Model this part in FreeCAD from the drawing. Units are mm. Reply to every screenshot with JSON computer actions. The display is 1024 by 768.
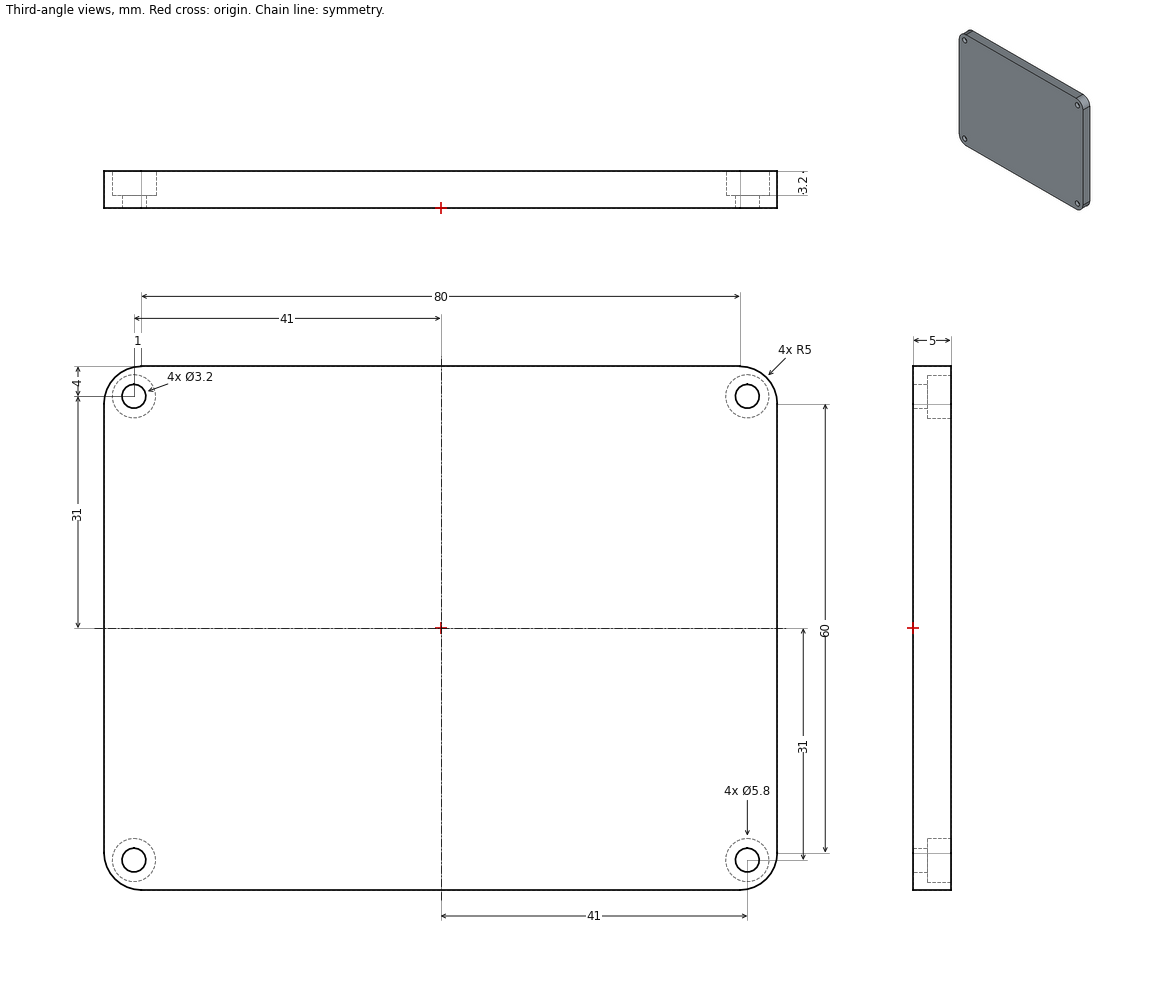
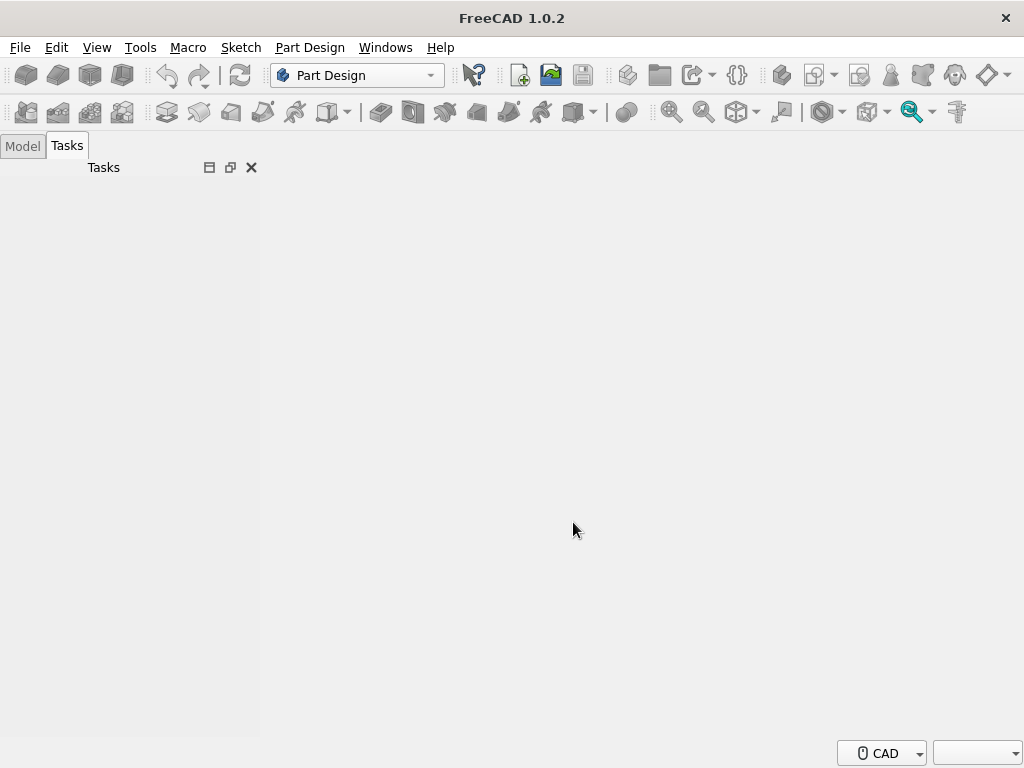
{"action": "key", "text": "ctrl+n"}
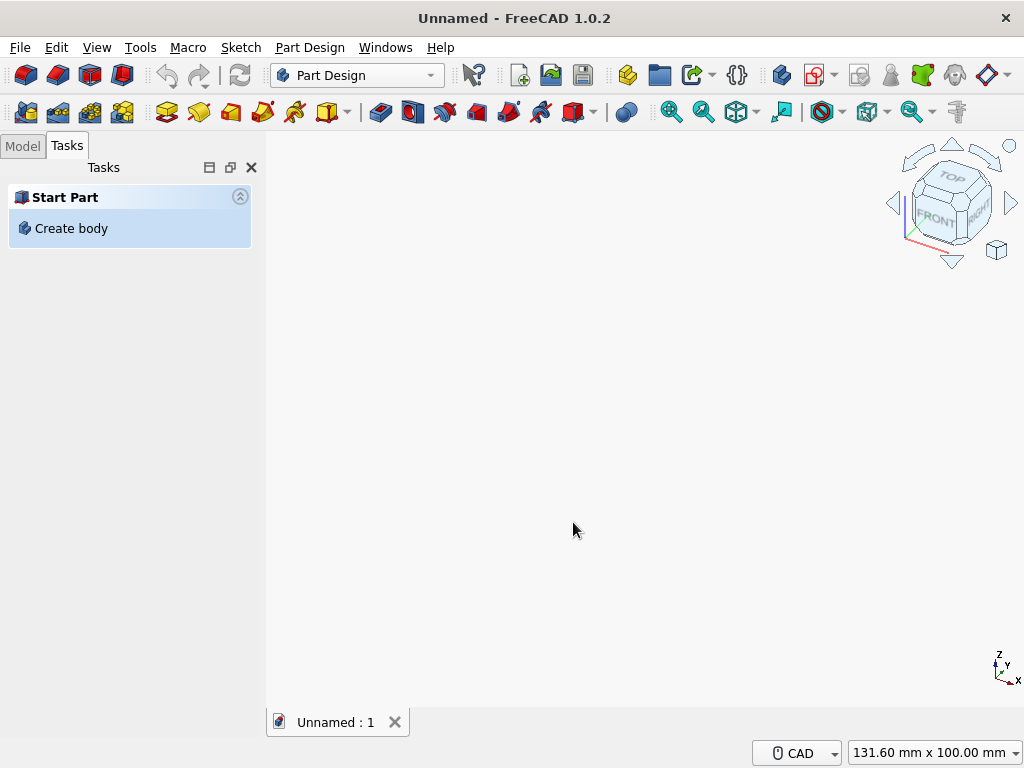
{"action": "left_click", "coordinate": [814, 76]}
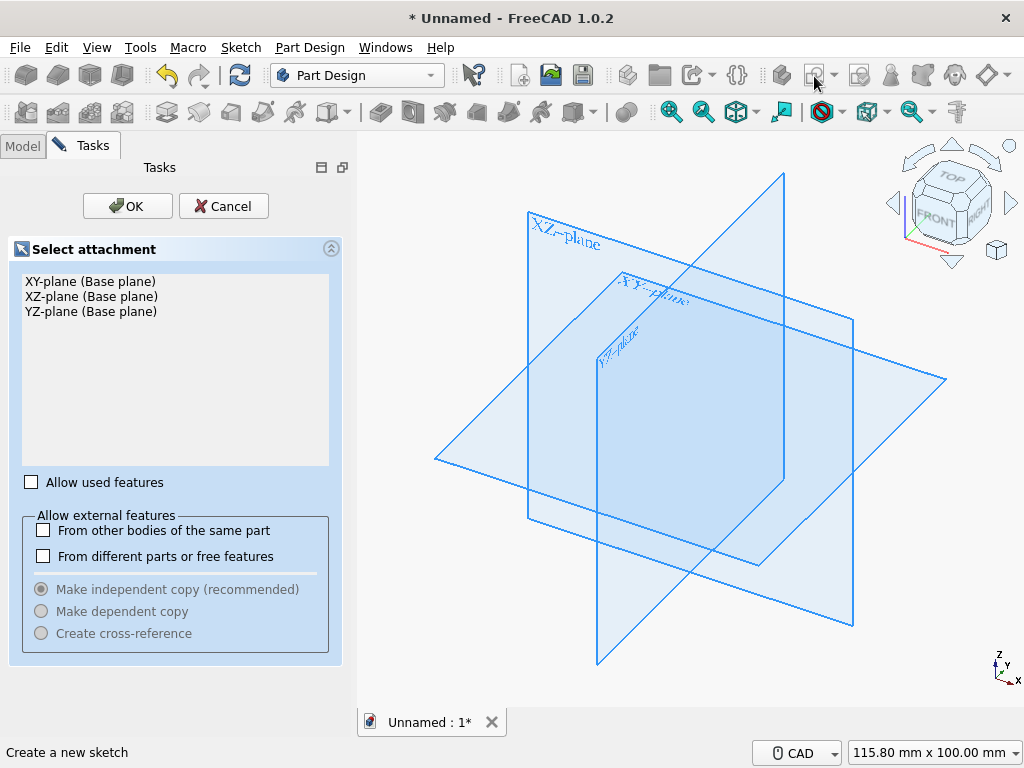
{"action": "left_click", "coordinate": [82, 296]}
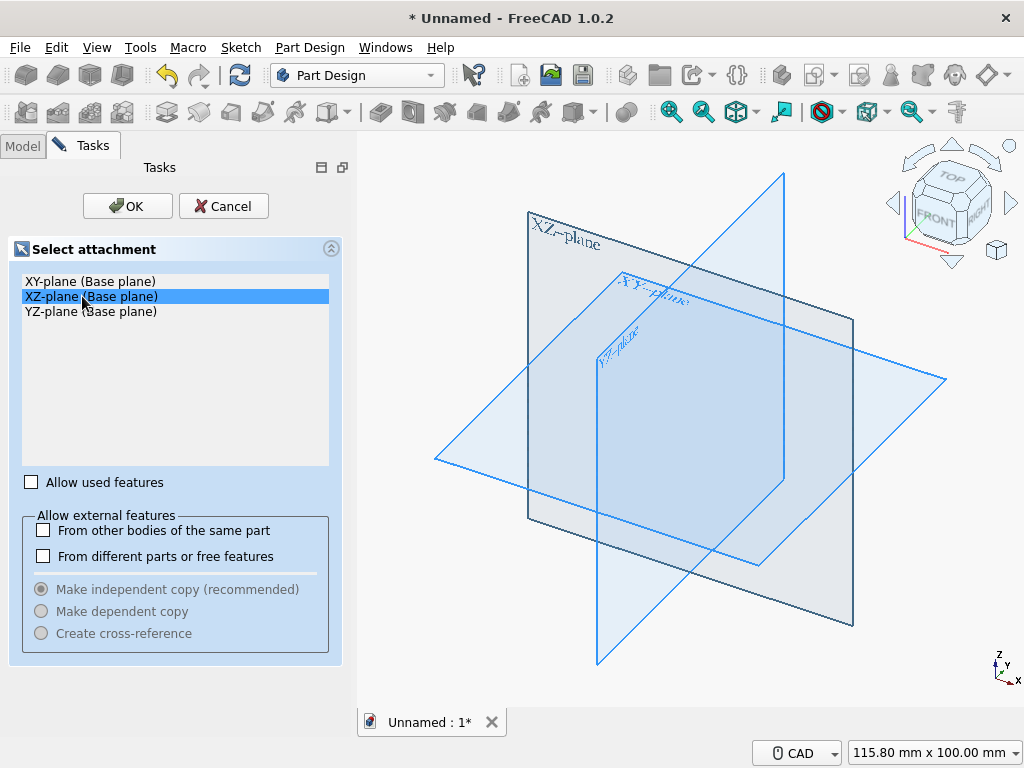
{"action": "left_click", "coordinate": [128, 206]}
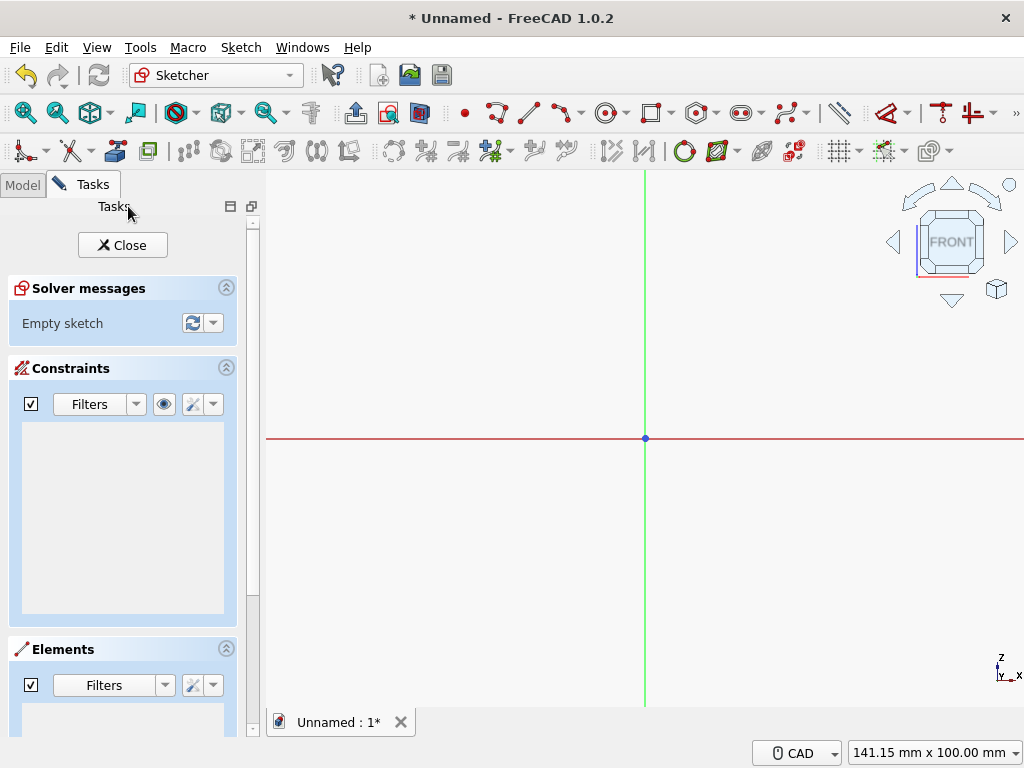
{"action": "scroll", "coordinate": [294, 439], "scroll_direction": "down", "scroll_amount": 1}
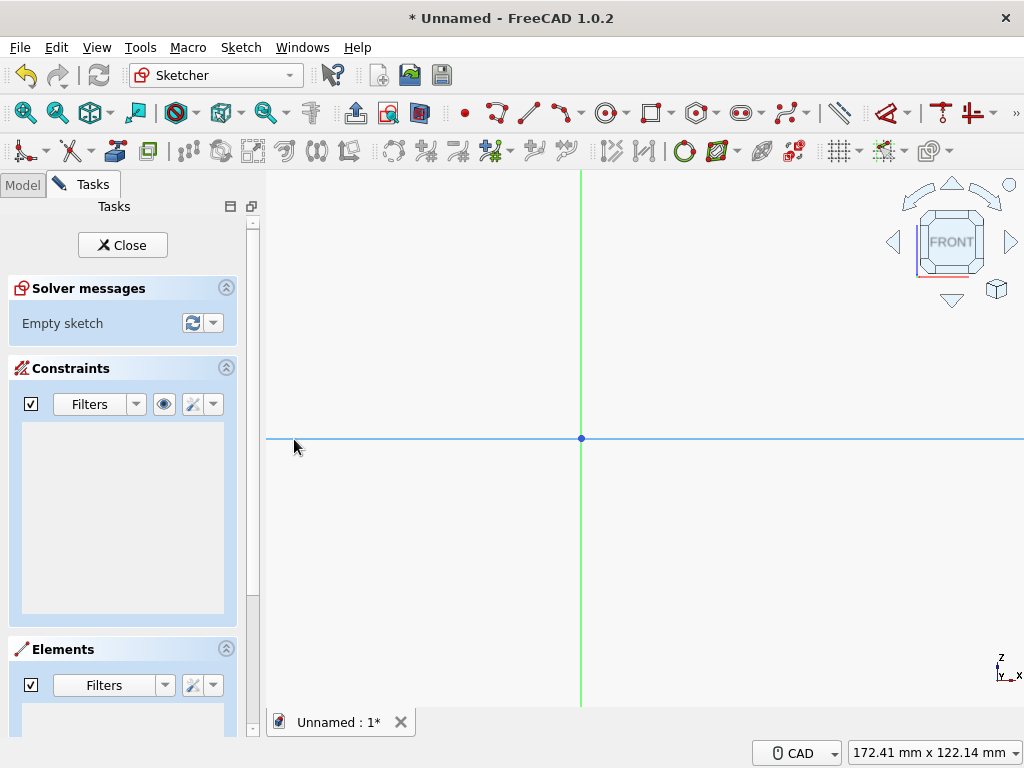
{"action": "key", "text": "g l"}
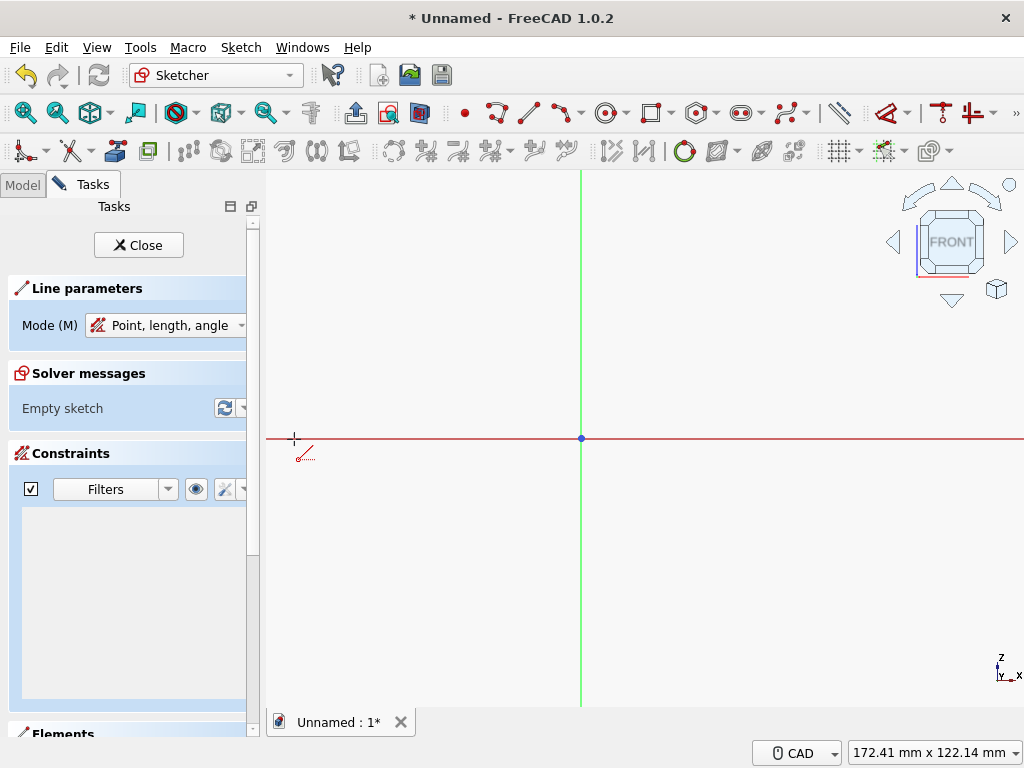
{"action": "left_click", "coordinate": [406, 285]}
{"action": "left_click", "coordinate": [757, 285]}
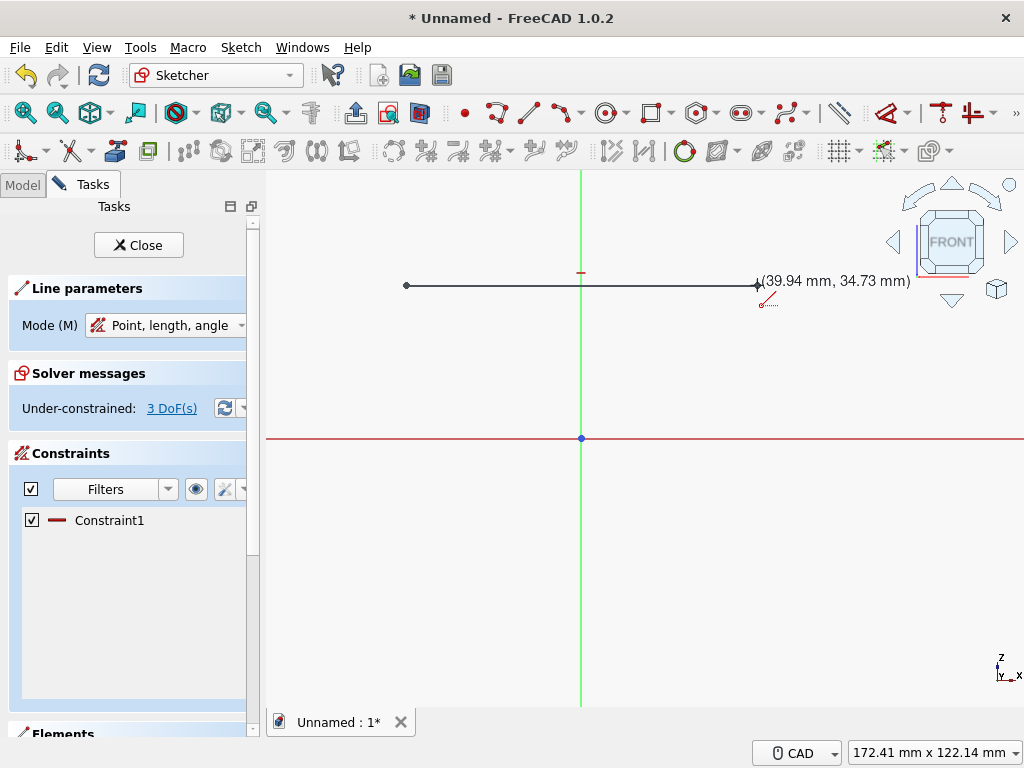
{"action": "left_click", "coordinate": [779, 307]}
{"action": "left_click", "coordinate": [779, 571]}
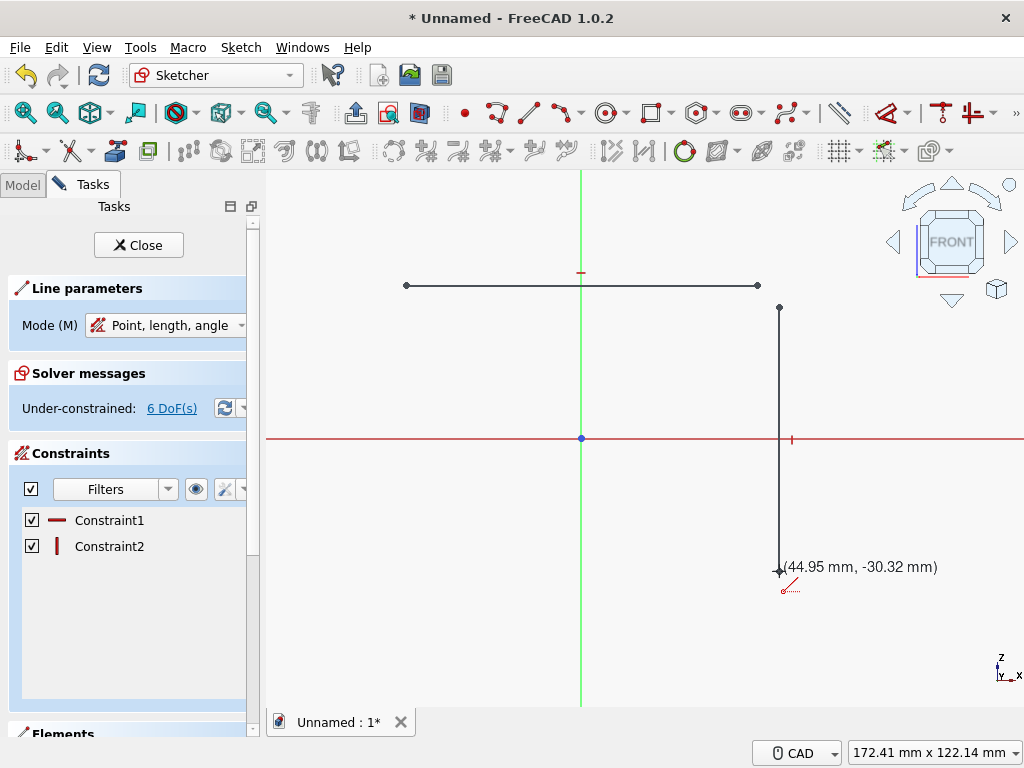
{"action": "left_click", "coordinate": [757, 593]}
{"action": "left_click", "coordinate": [406, 593]}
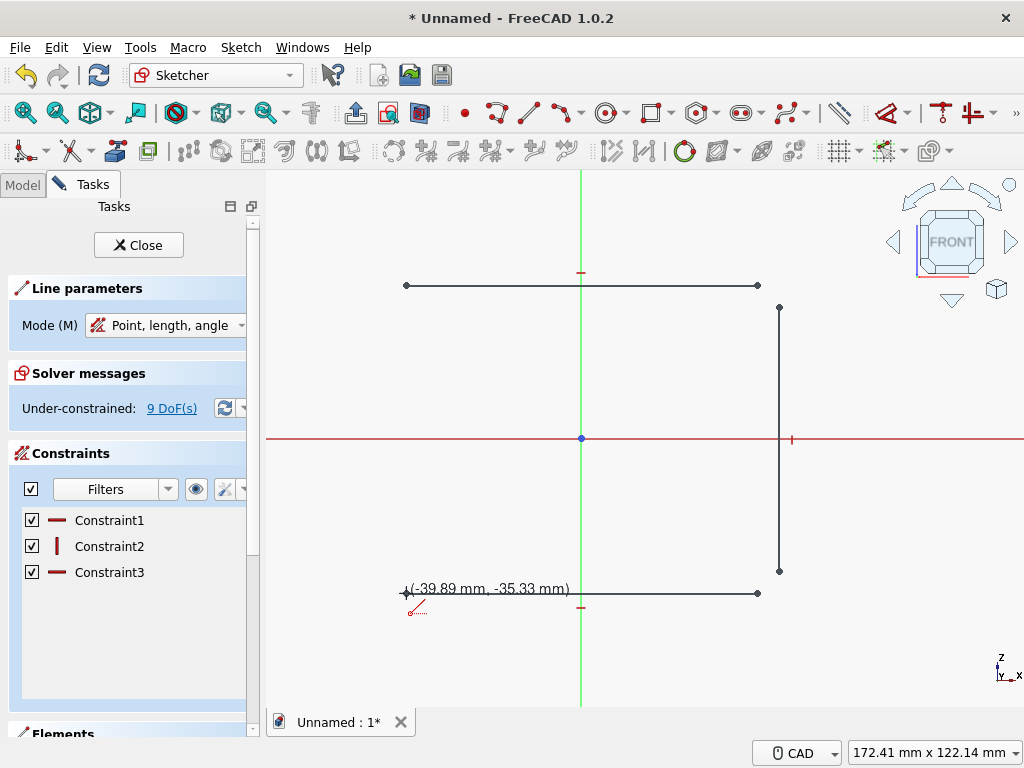
{"action": "left_click", "coordinate": [384, 571]}
{"action": "left_click", "coordinate": [384, 307]}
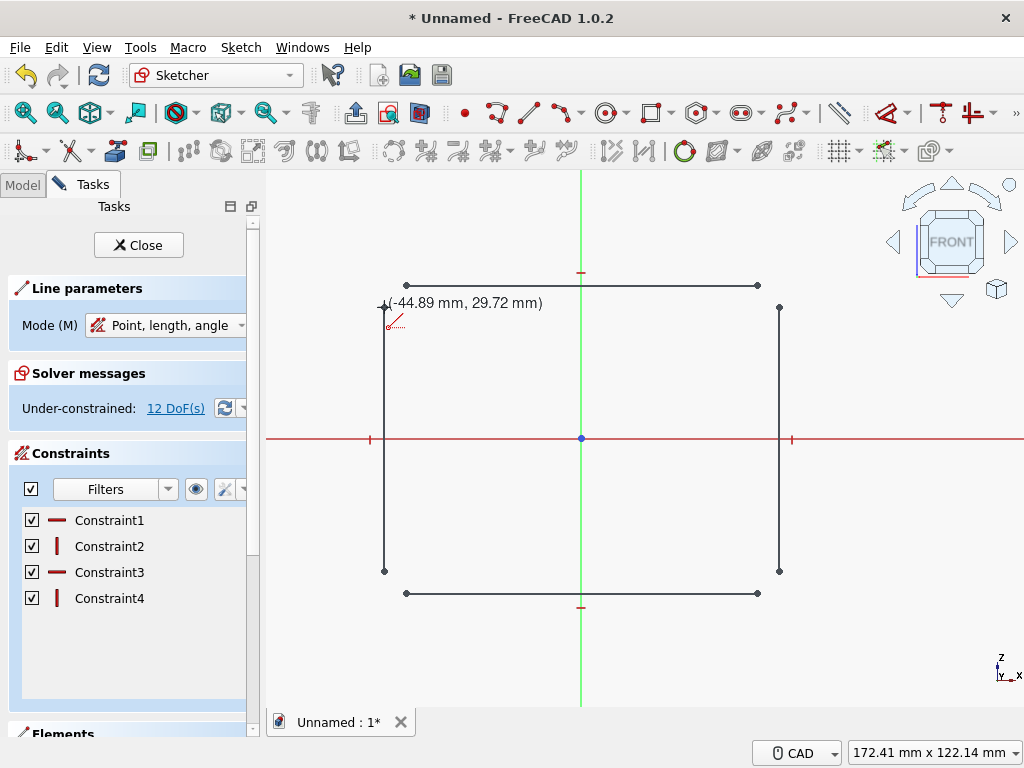
{"action": "left_click", "coordinate": [562, 114]}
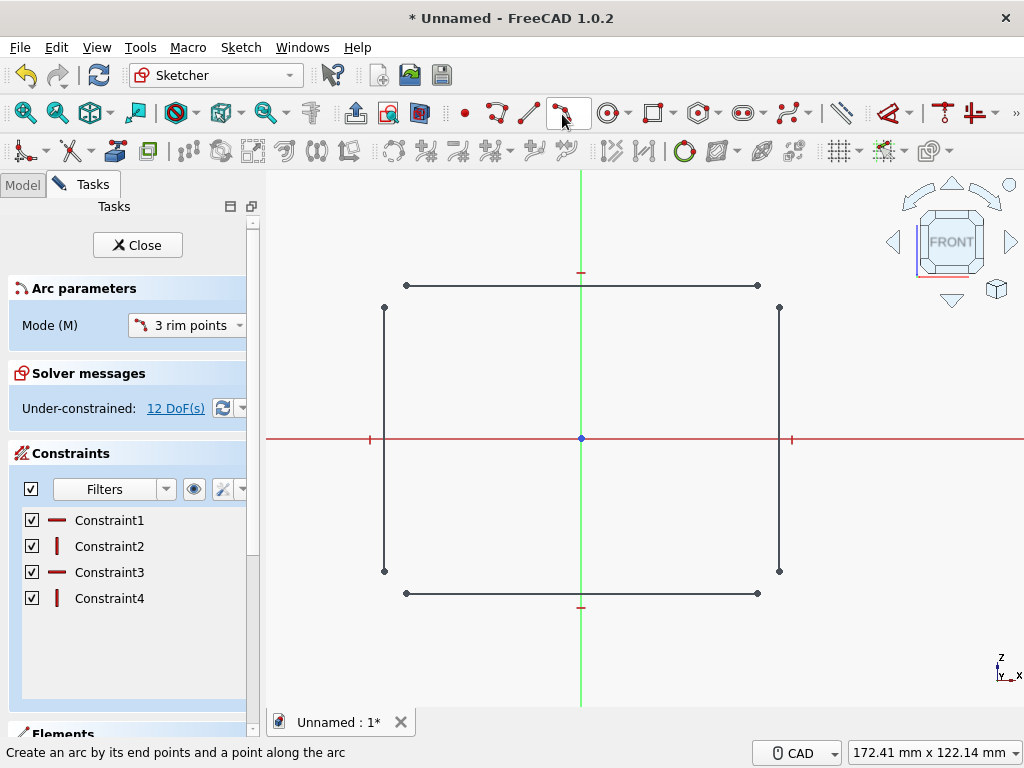
{"action": "left_click", "coordinate": [757, 286]}
{"action": "left_click", "coordinate": [779, 308]}